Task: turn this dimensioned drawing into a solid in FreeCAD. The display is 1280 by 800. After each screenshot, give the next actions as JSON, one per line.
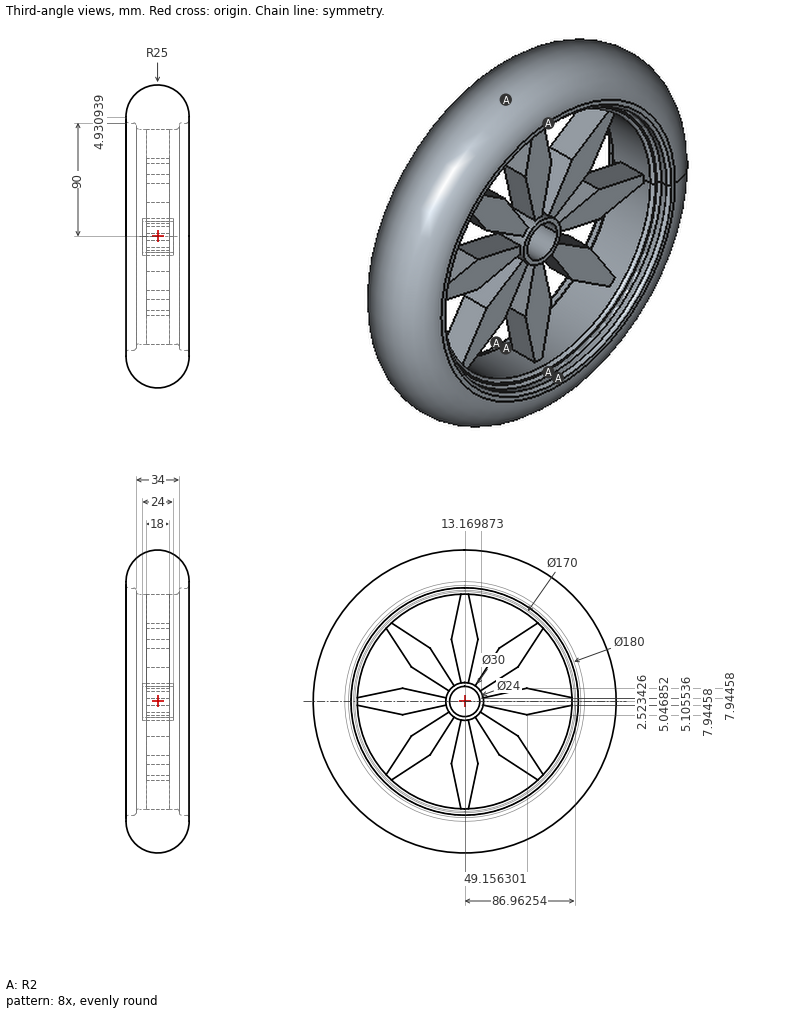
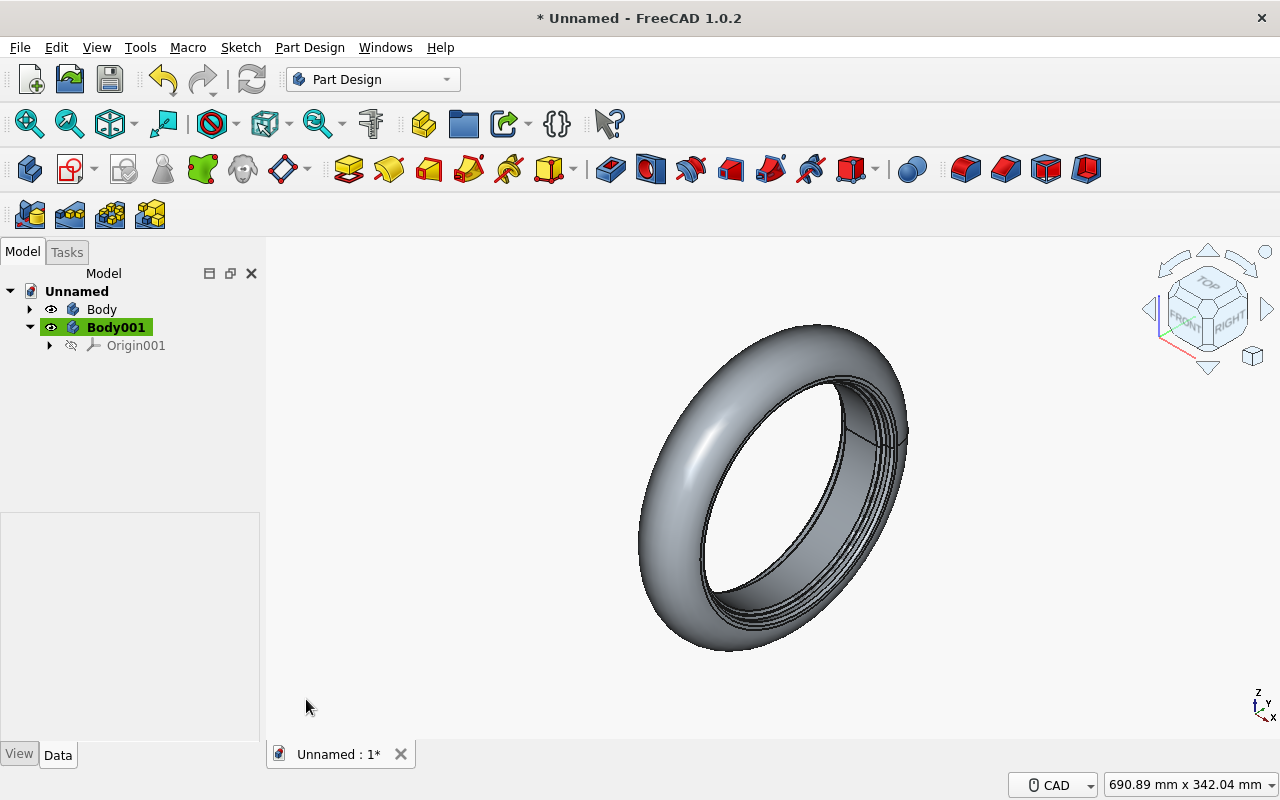
{"action": "left_click", "coordinate": [70, 170]}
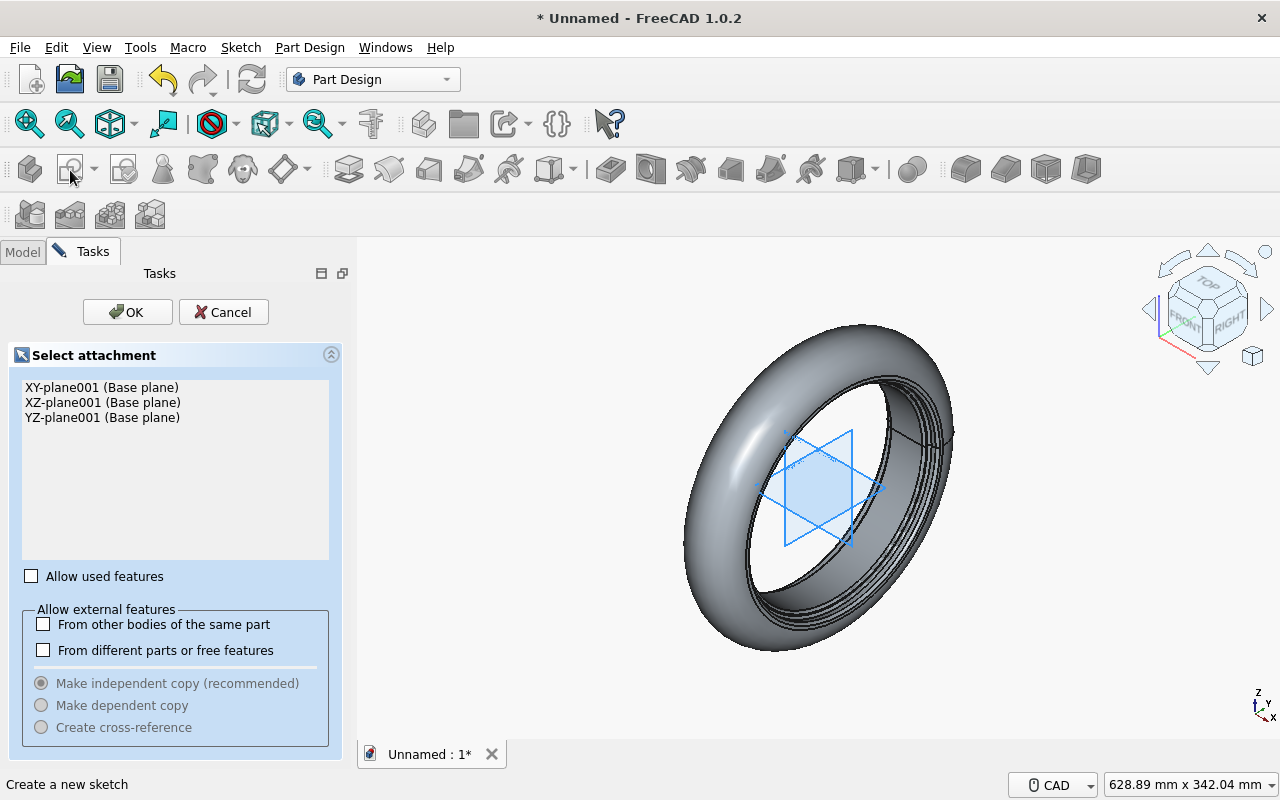
{"action": "left_click", "coordinate": [82, 418]}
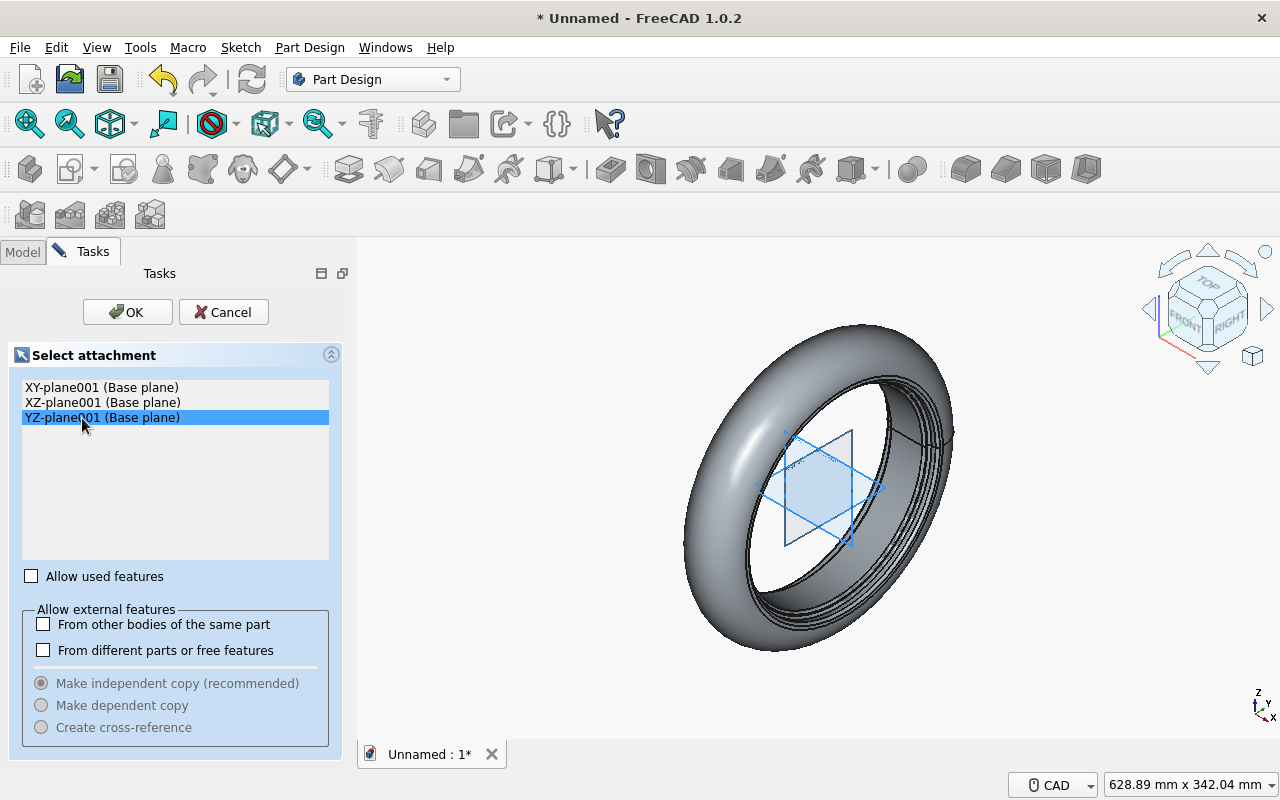
{"action": "left_click", "coordinate": [128, 312]}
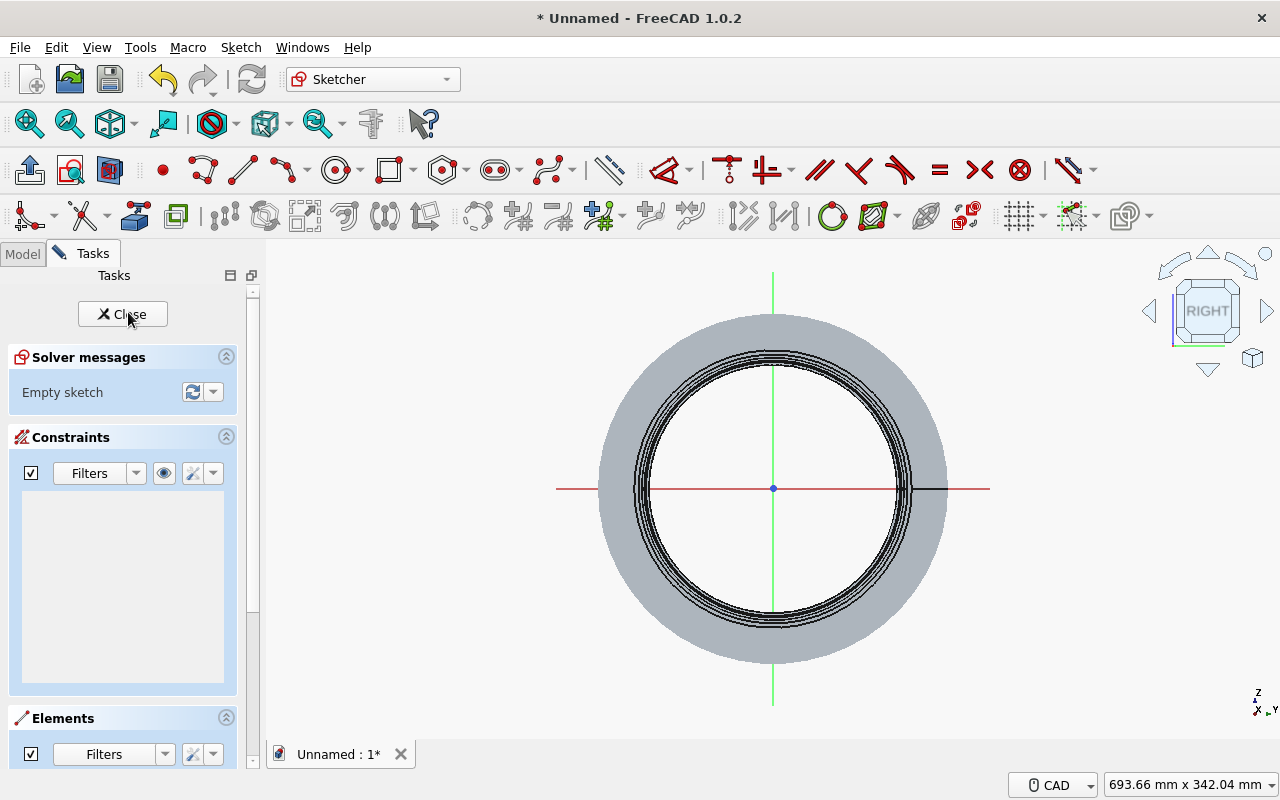
{"action": "scroll", "coordinate": [784, 489], "scroll_direction": "up", "scroll_amount": 10}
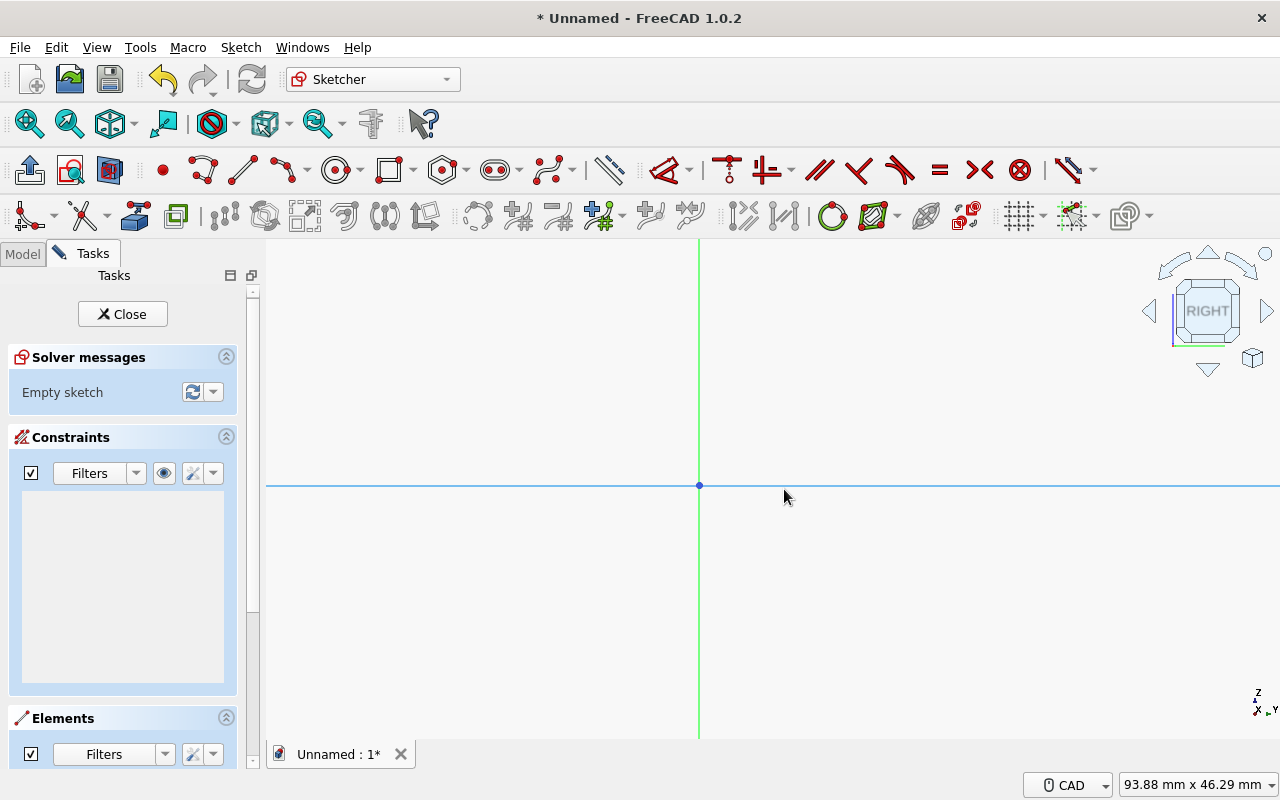
{"action": "key", "text": "g c"}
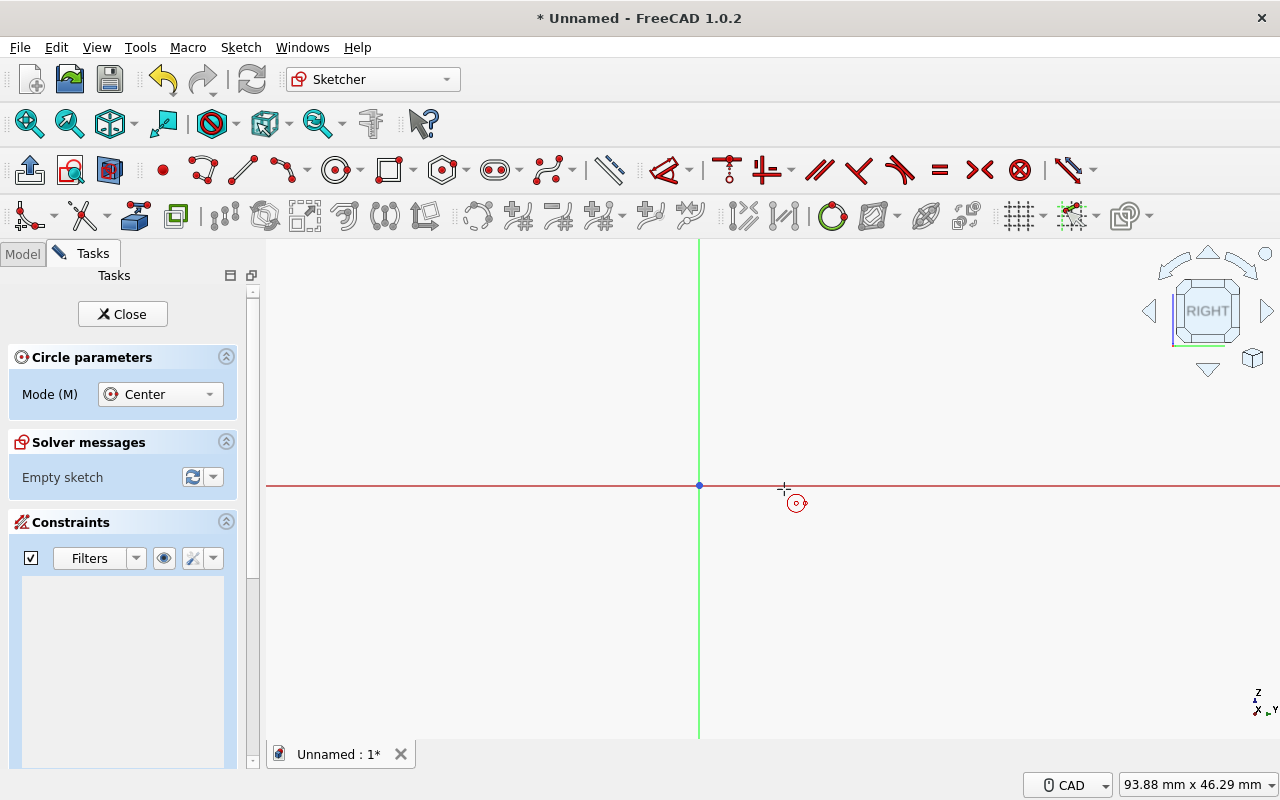
{"action": "left_click", "coordinate": [699, 486]}
{"action": "left_click", "coordinate": [814, 371]}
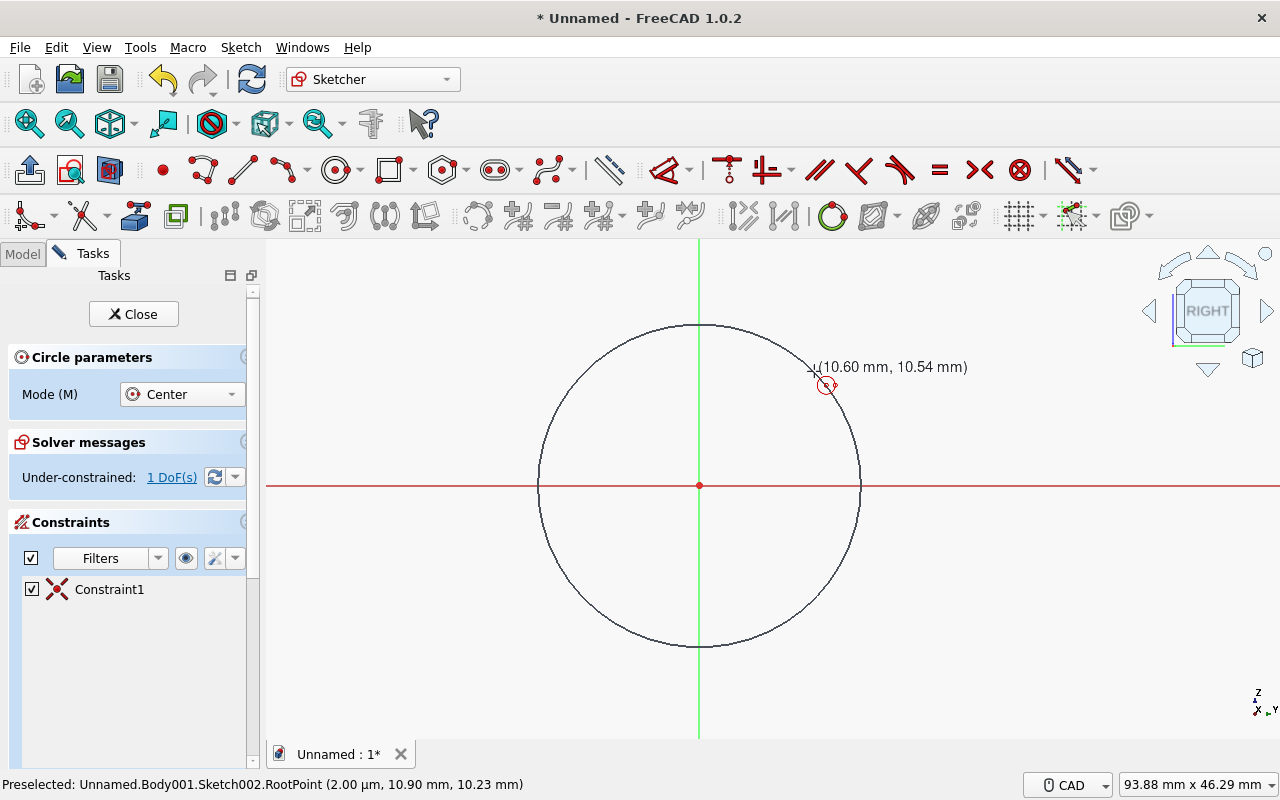
{"action": "left_click", "coordinate": [699, 486]}
{"action": "left_click", "coordinate": [791, 394]}
{"action": "key", "text": "Escape"}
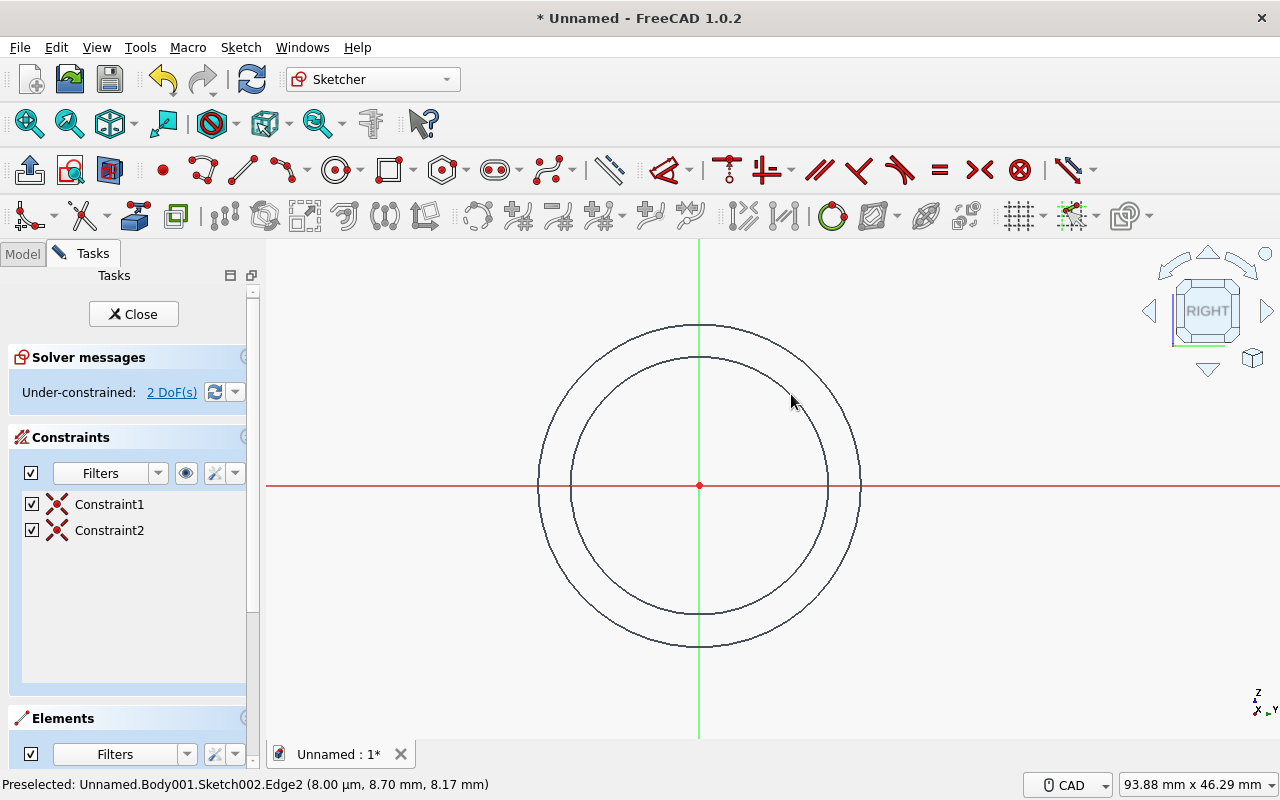
{"action": "key", "text": "d"}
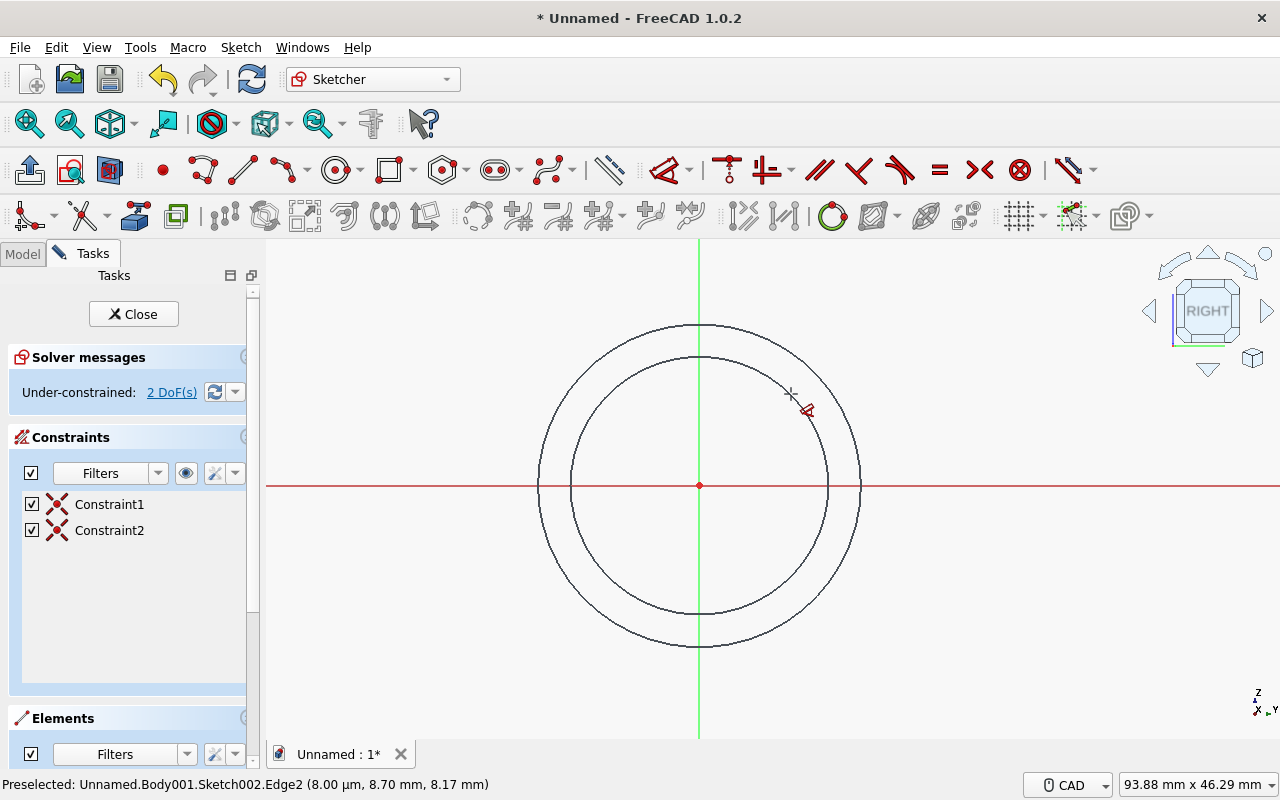
{"action": "left_click", "coordinate": [813, 371]}
{"action": "left_click", "coordinate": [836, 348]}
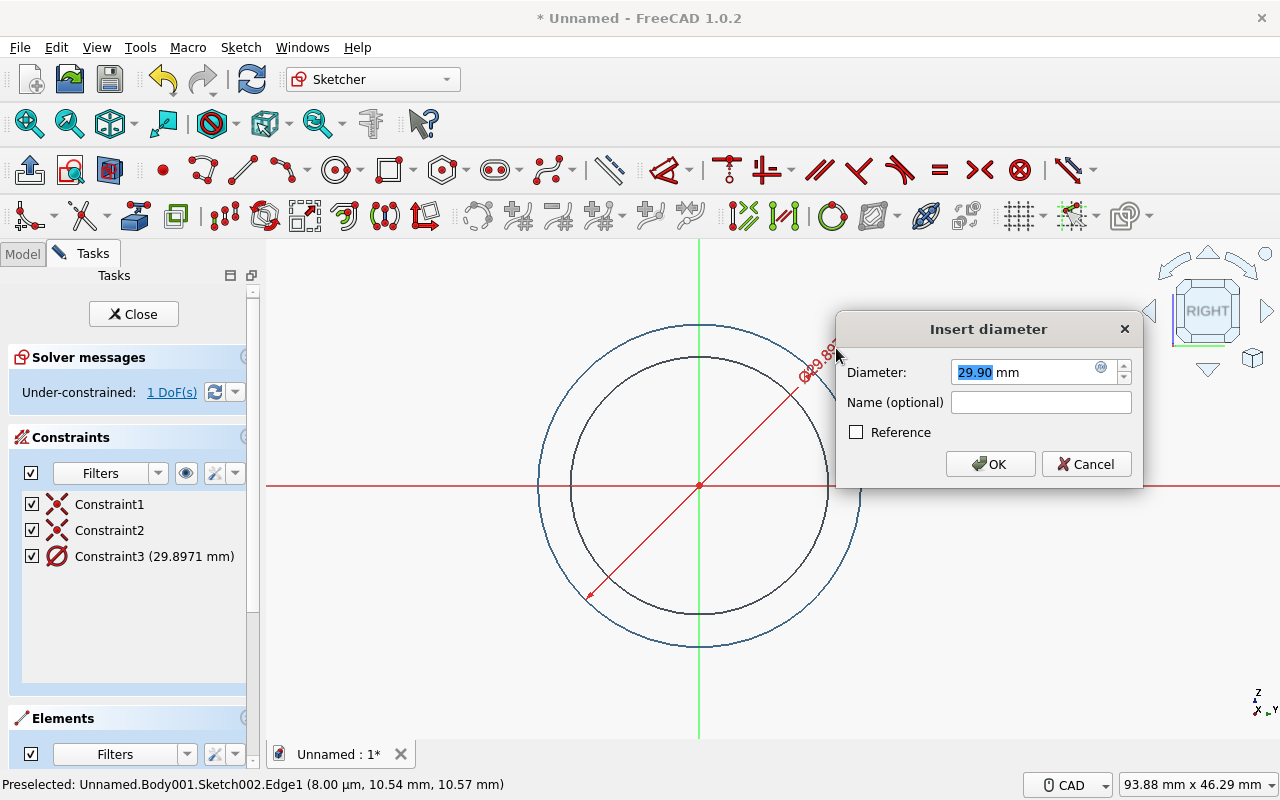
{"action": "type", "text": "30"}
{"action": "key", "text": "Return"}